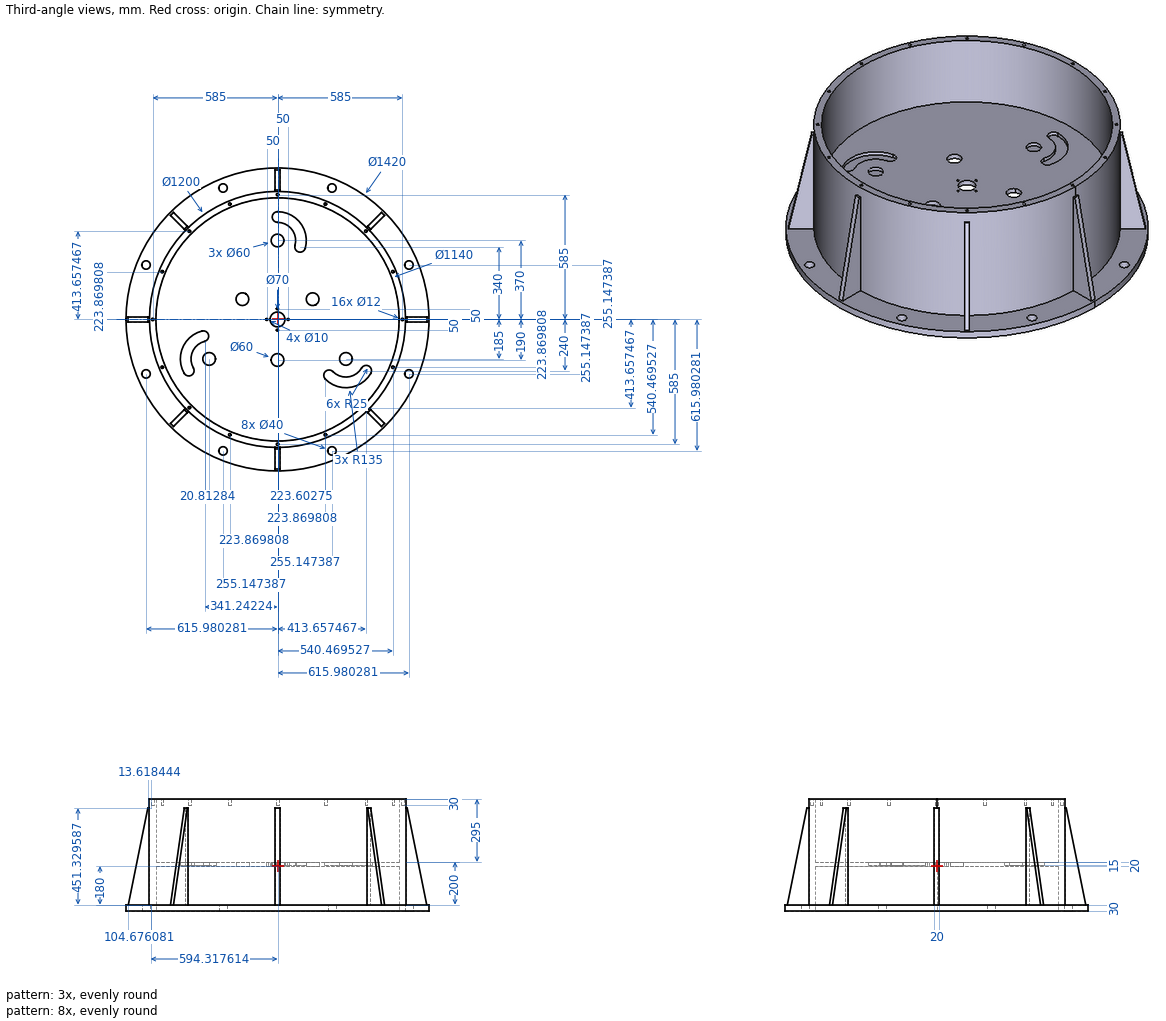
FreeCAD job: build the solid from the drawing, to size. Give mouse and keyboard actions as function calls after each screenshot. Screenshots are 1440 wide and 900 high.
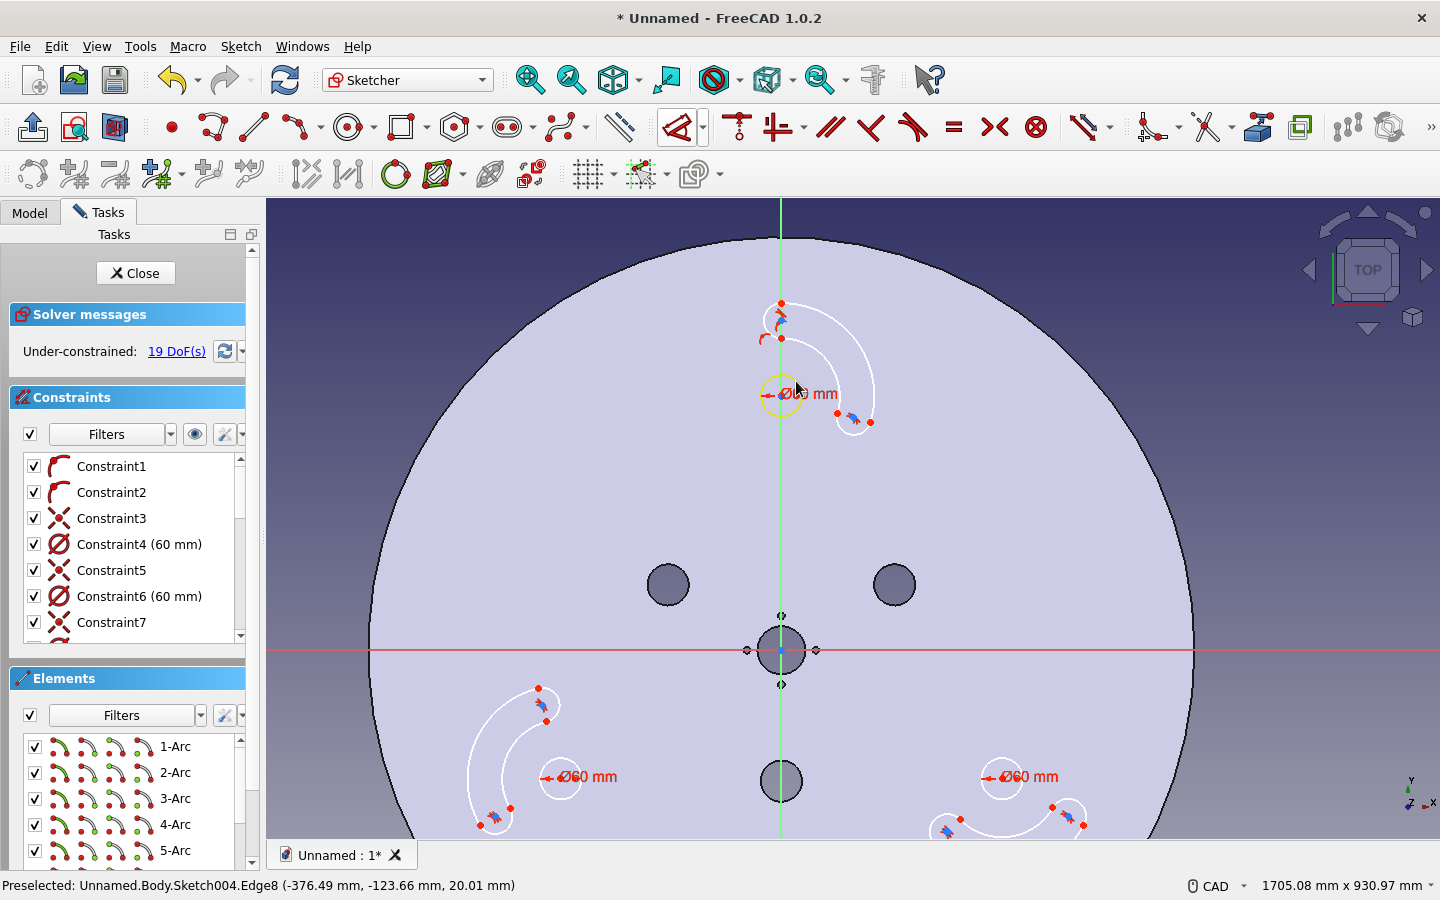
click(796, 381)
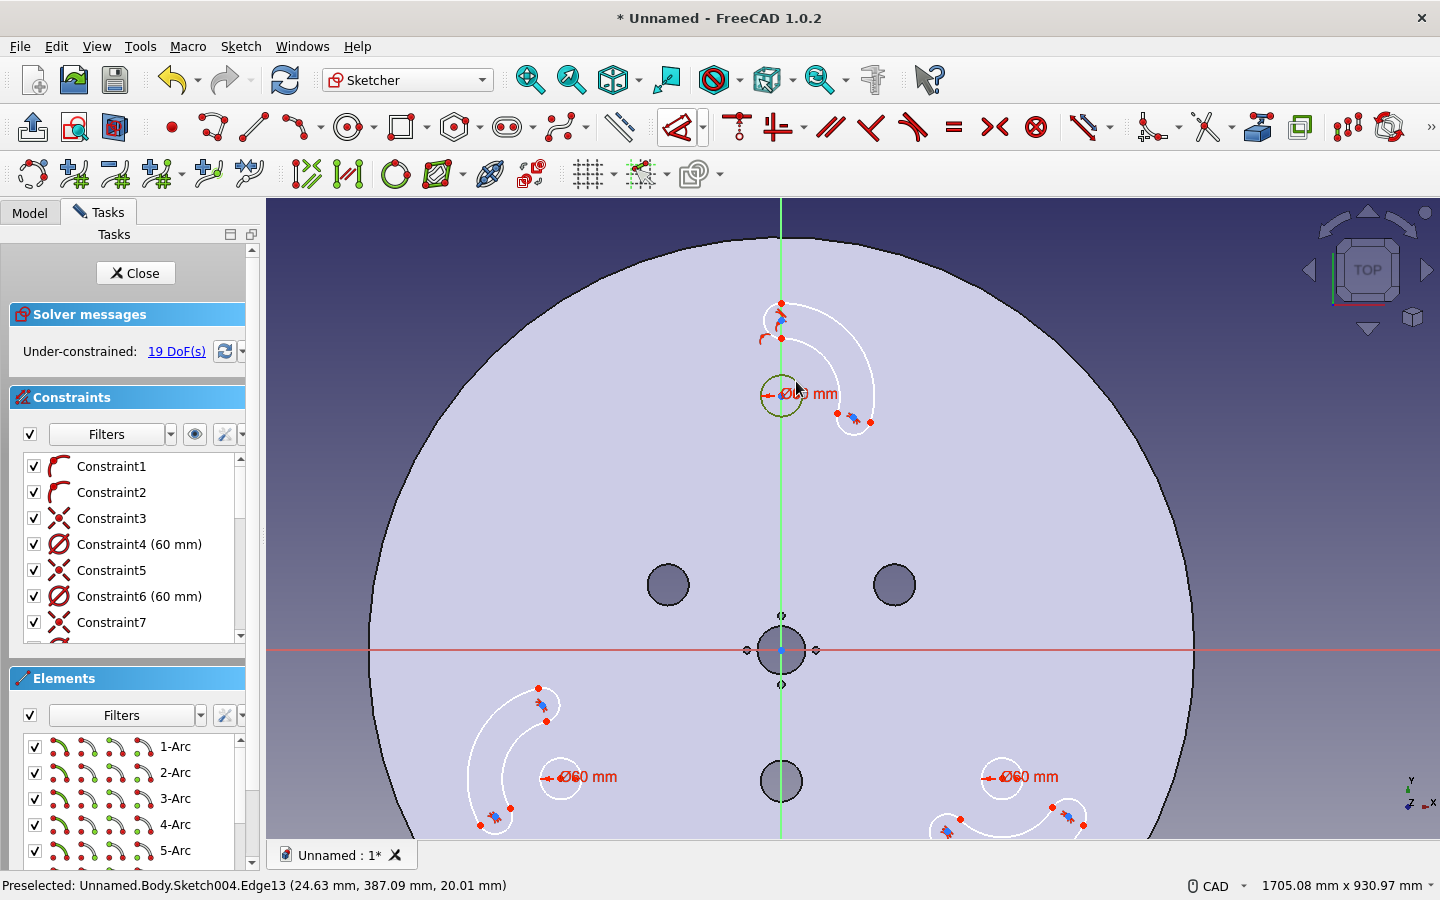
click(838, 381)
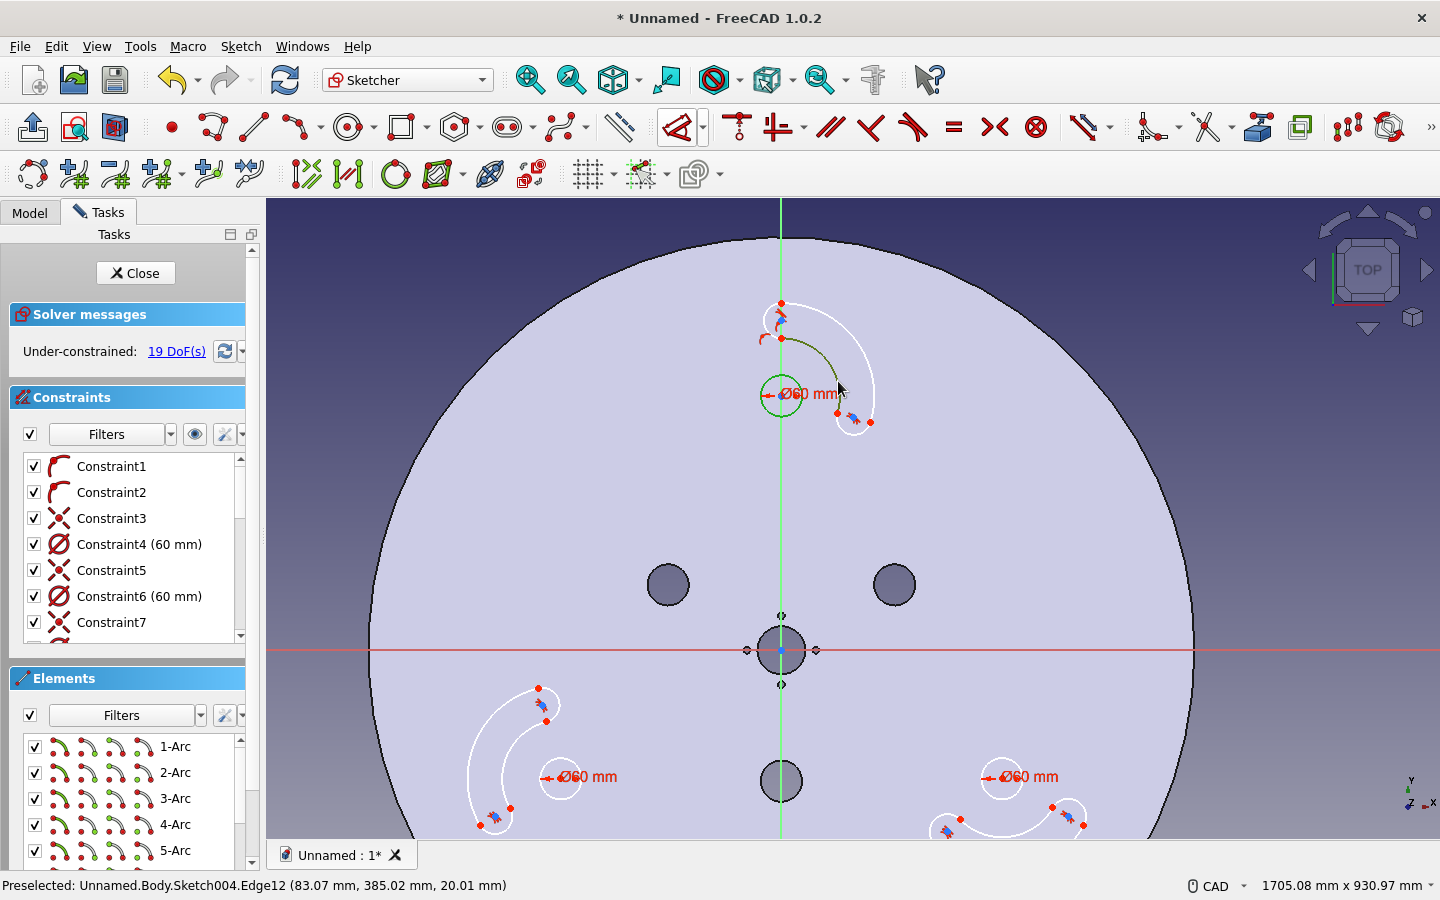
key(c)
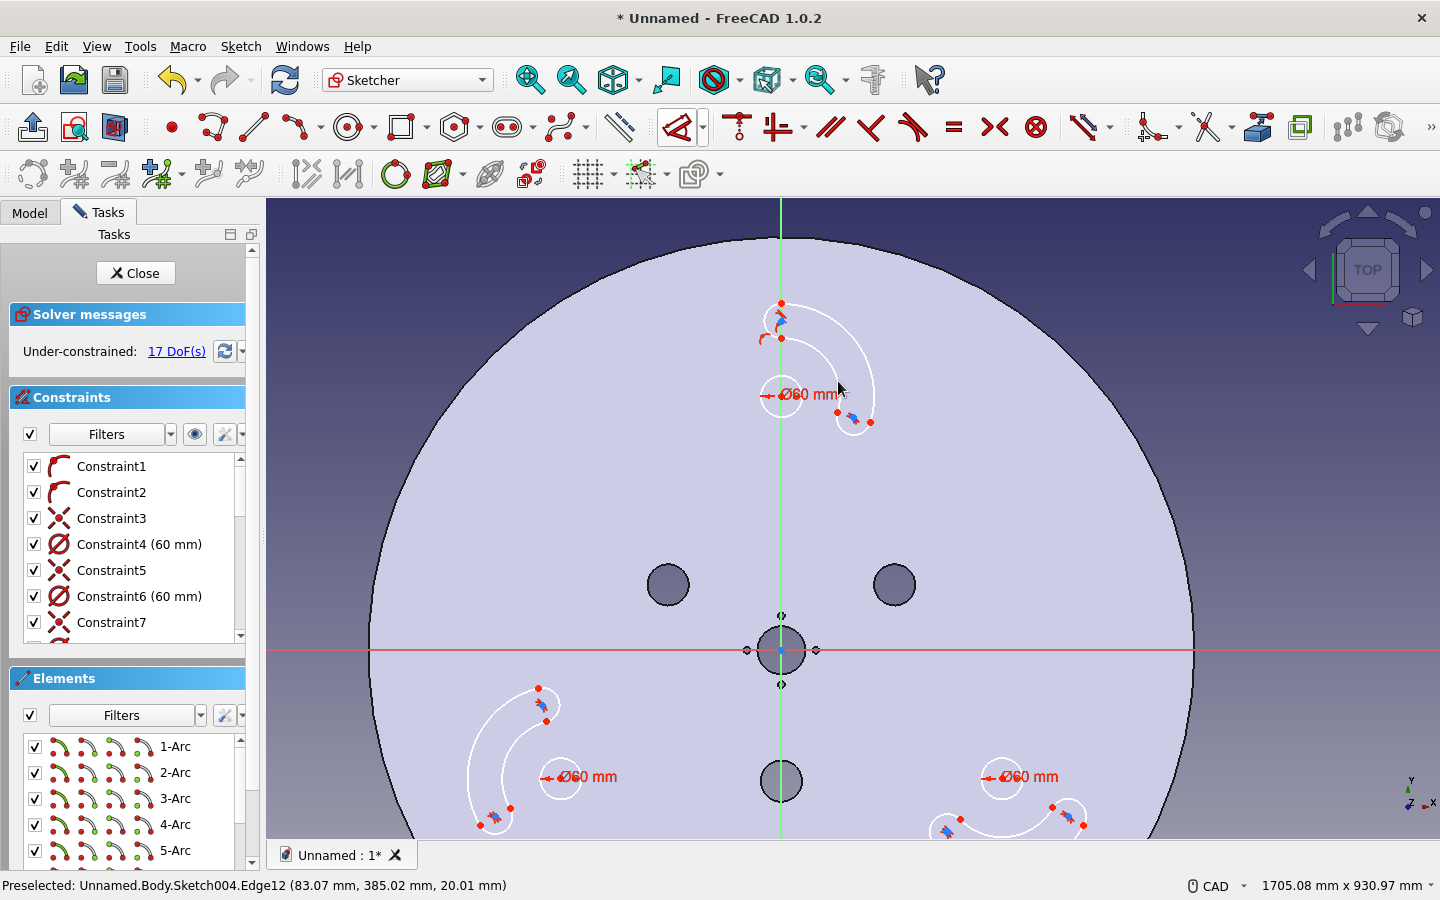
scroll(796, 381, down, 2)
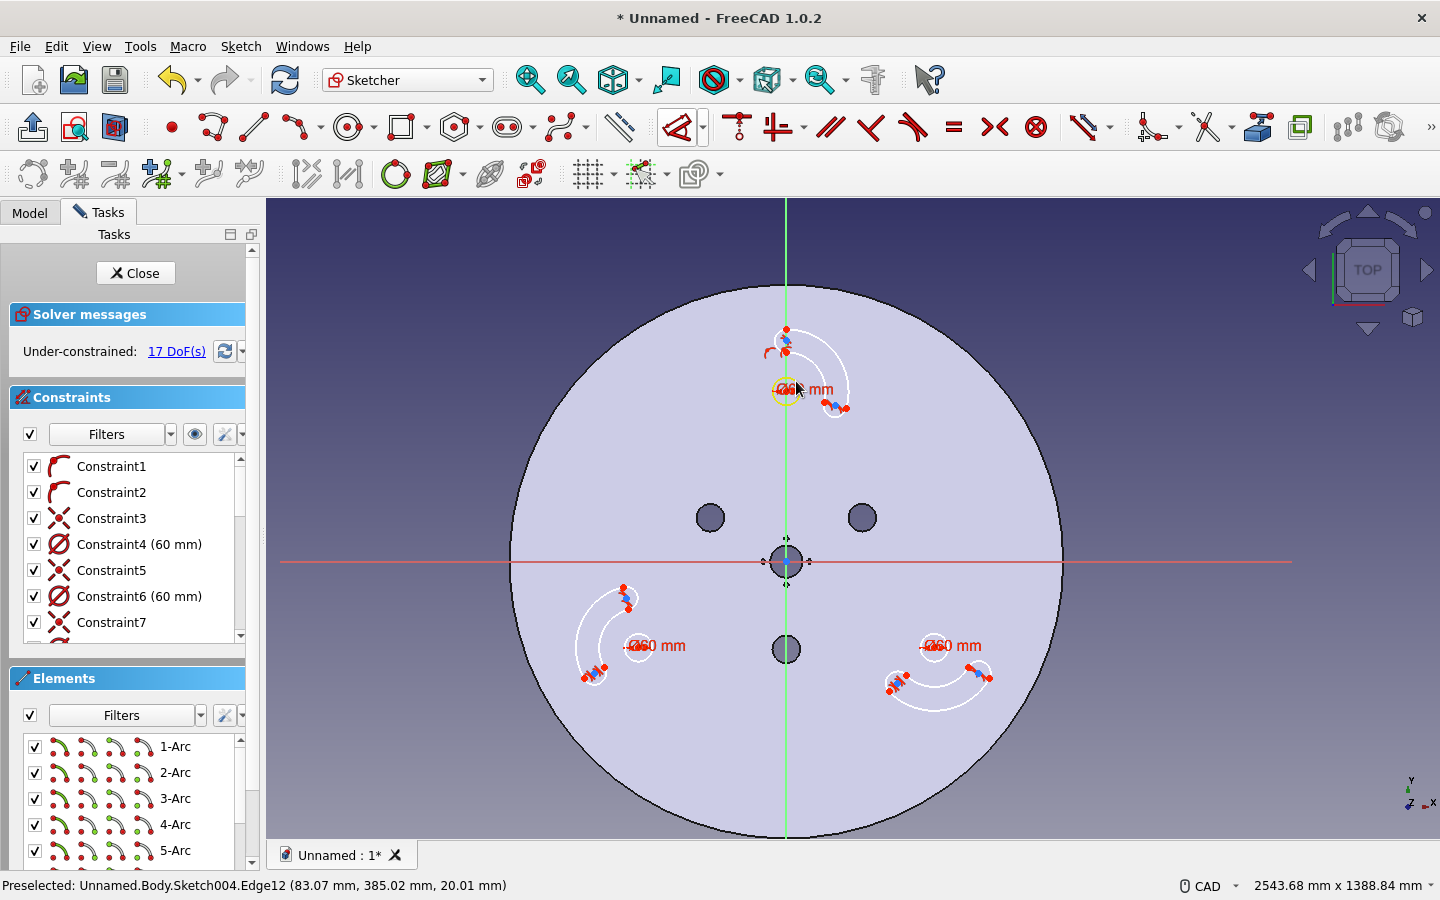
scroll(896, 672, up, 2)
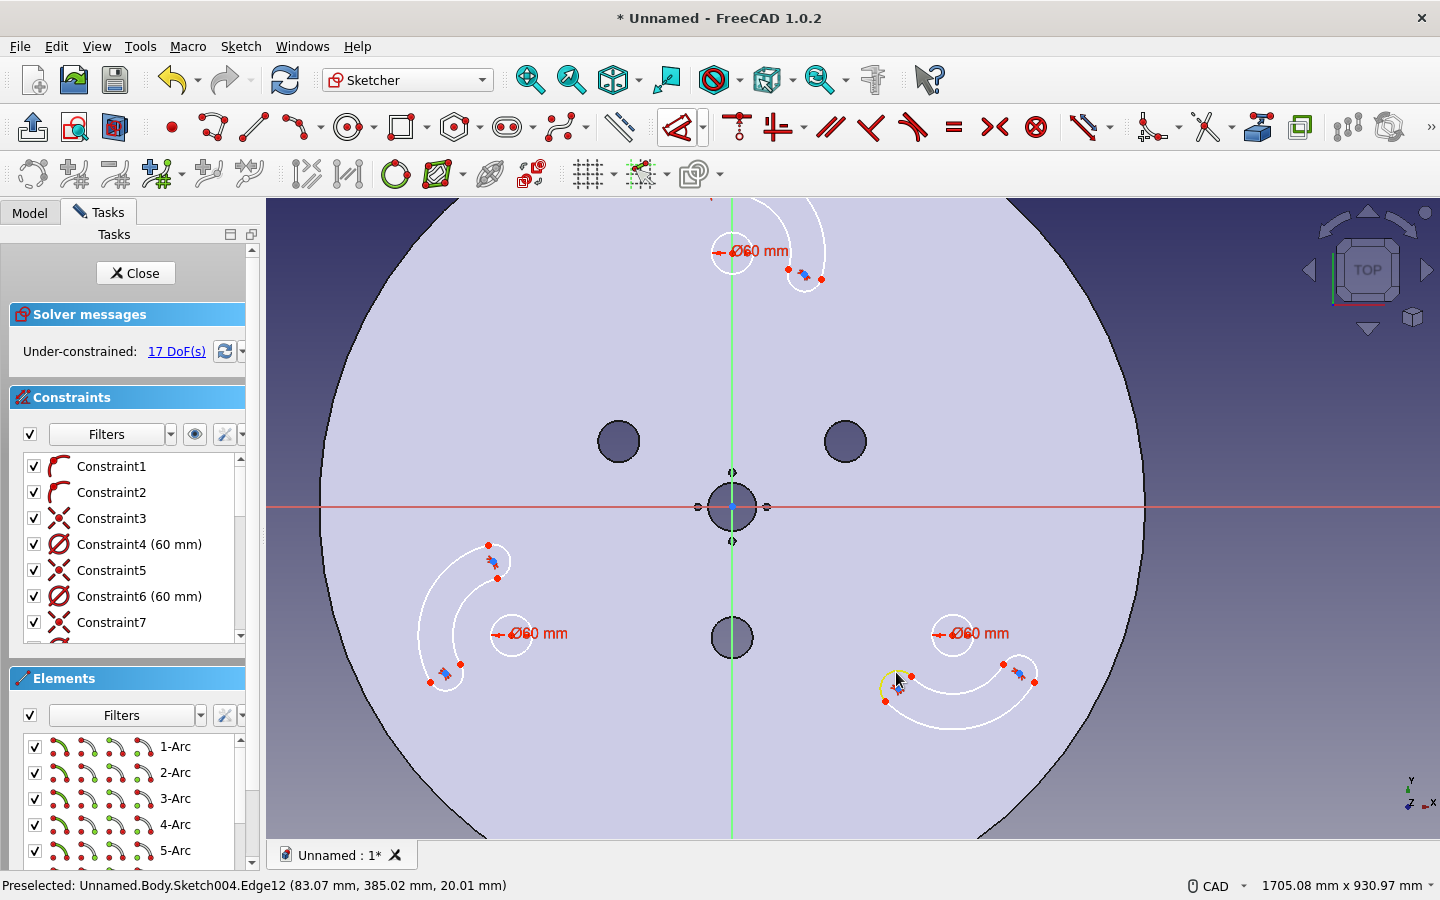
click(896, 671)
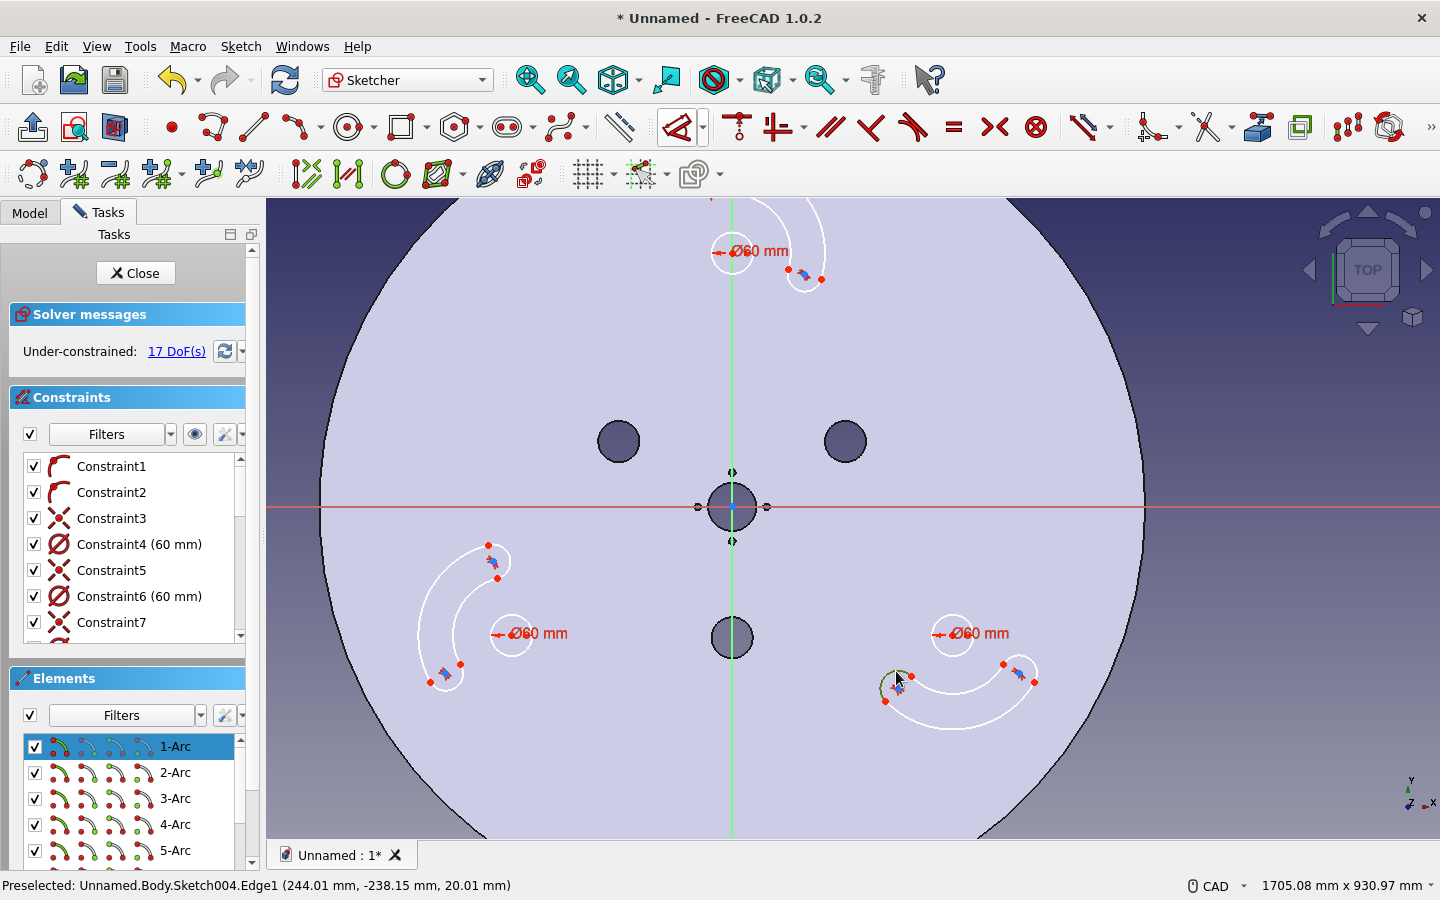
click(509, 568)